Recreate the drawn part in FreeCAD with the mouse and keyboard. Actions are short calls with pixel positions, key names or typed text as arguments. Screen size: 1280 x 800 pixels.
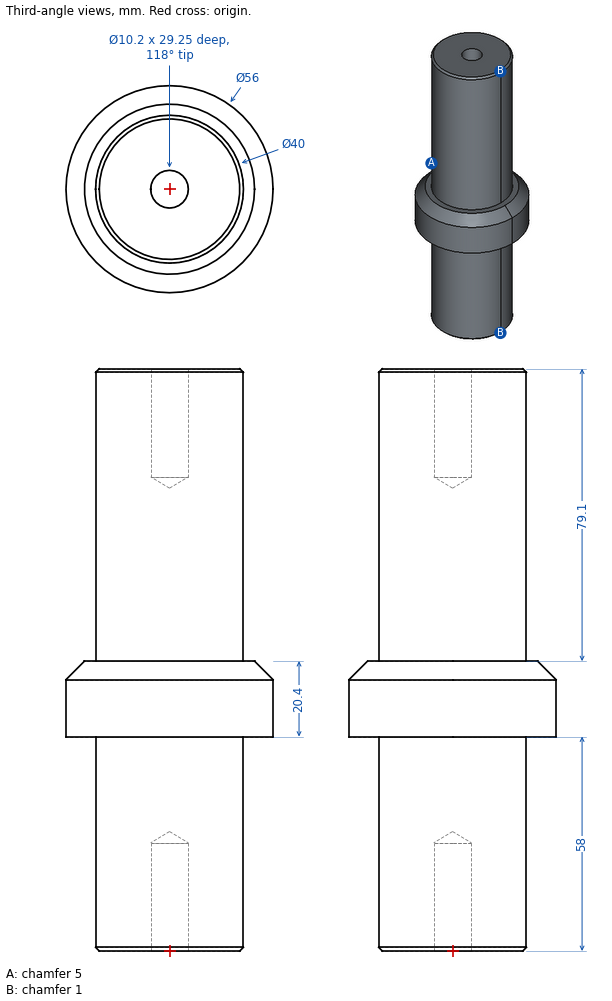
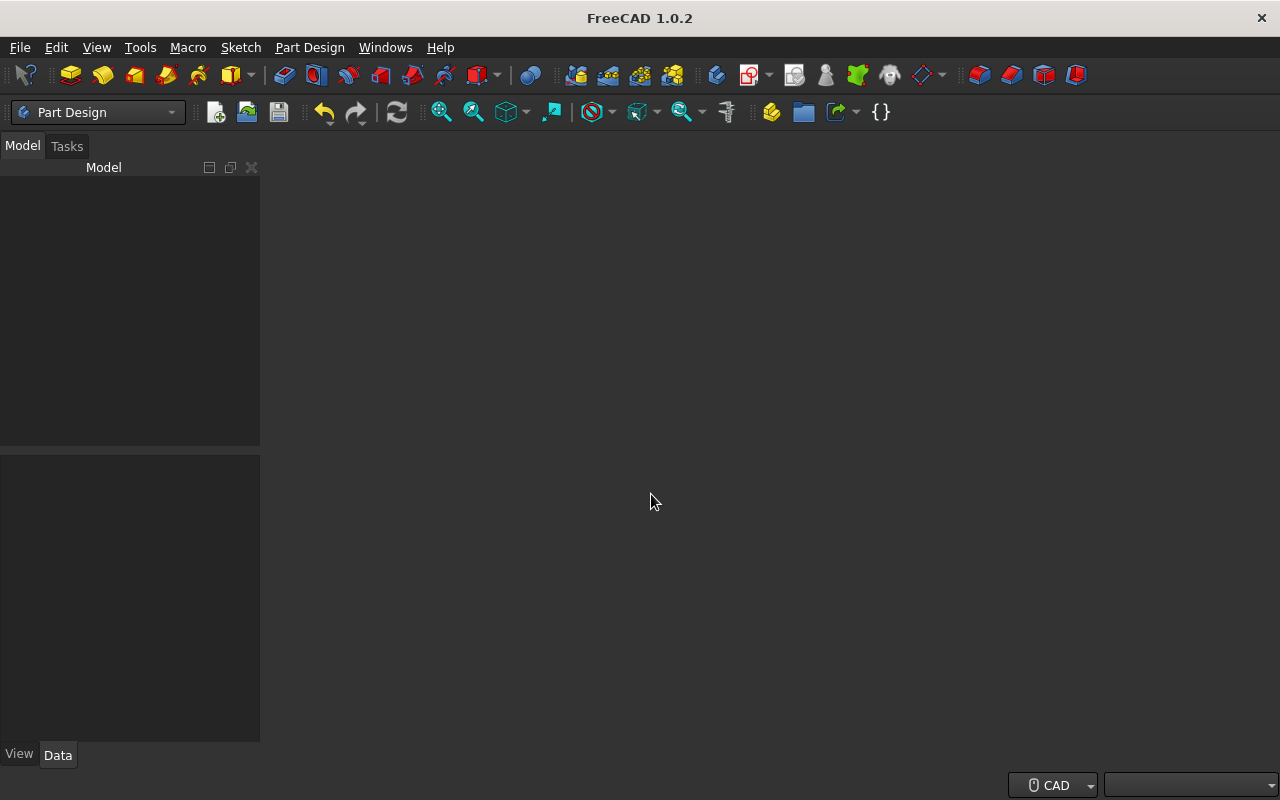
click(216, 112)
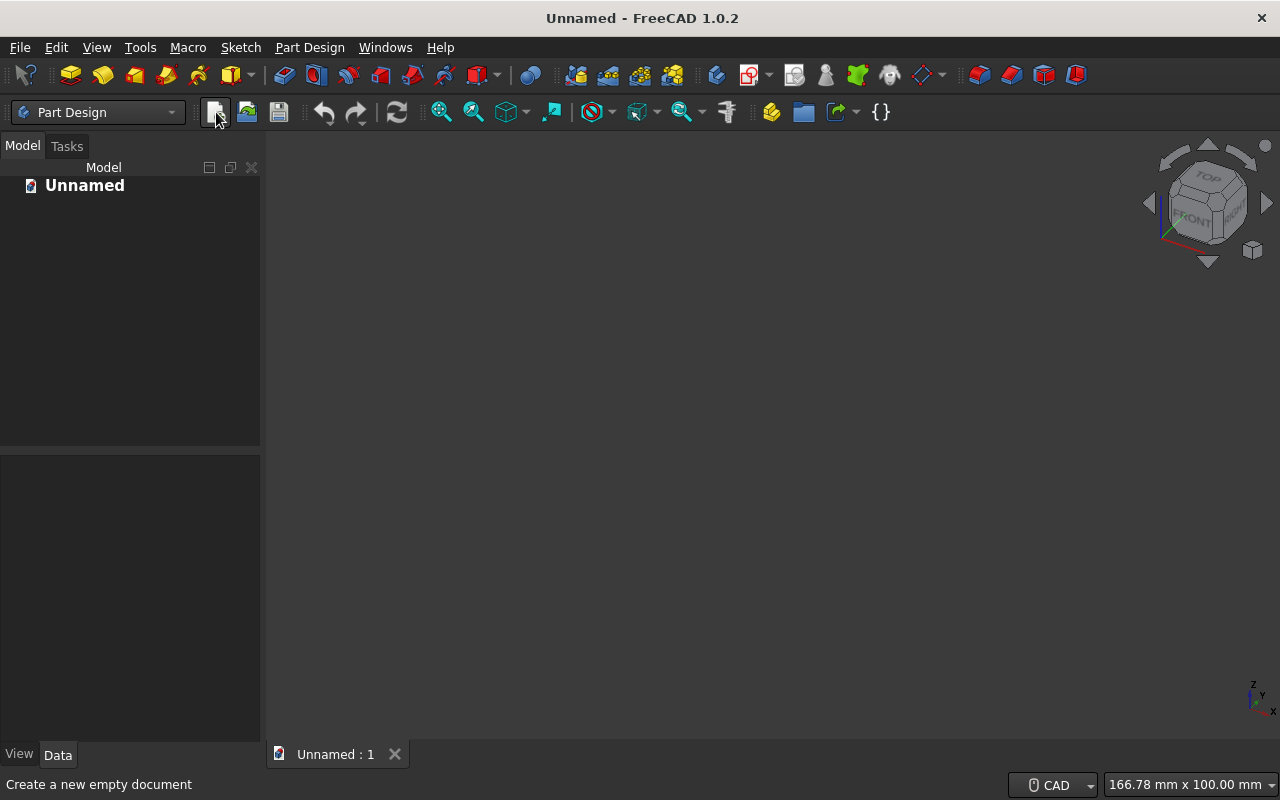
click(750, 76)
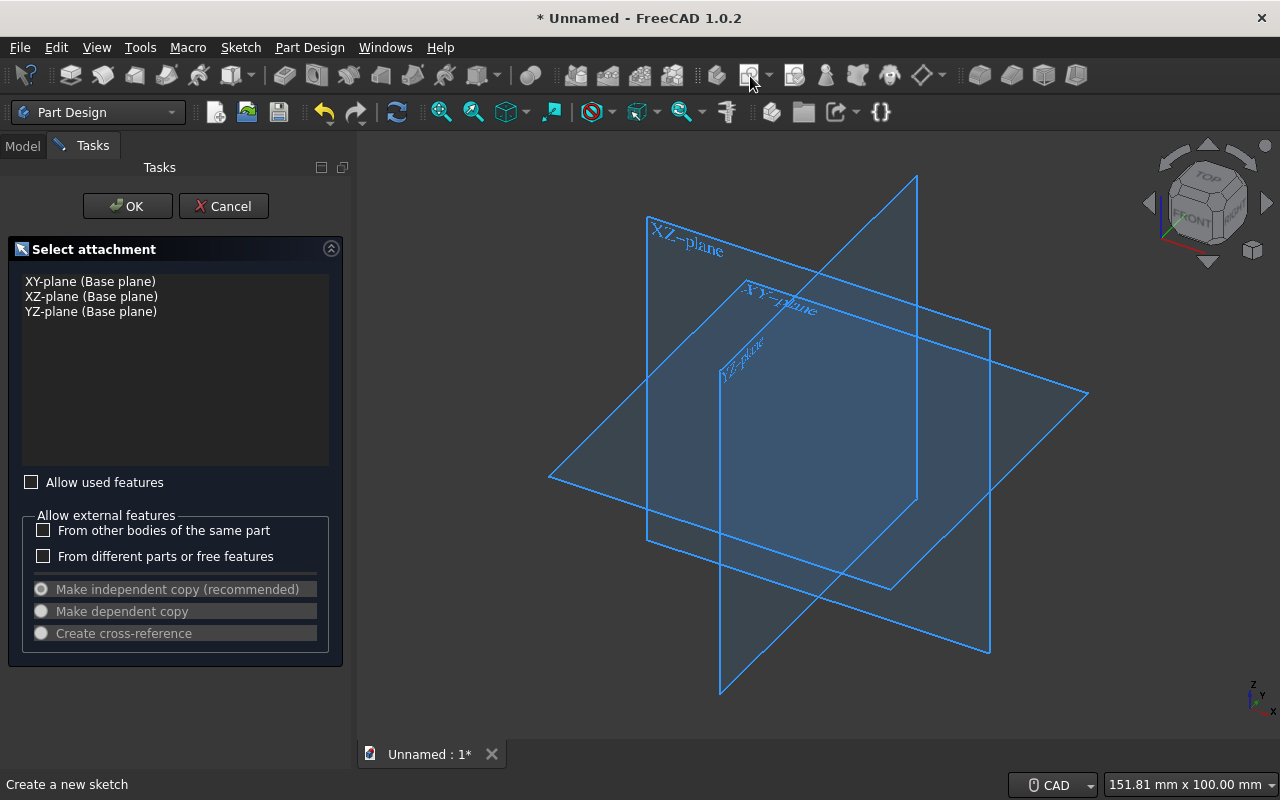
click(82, 282)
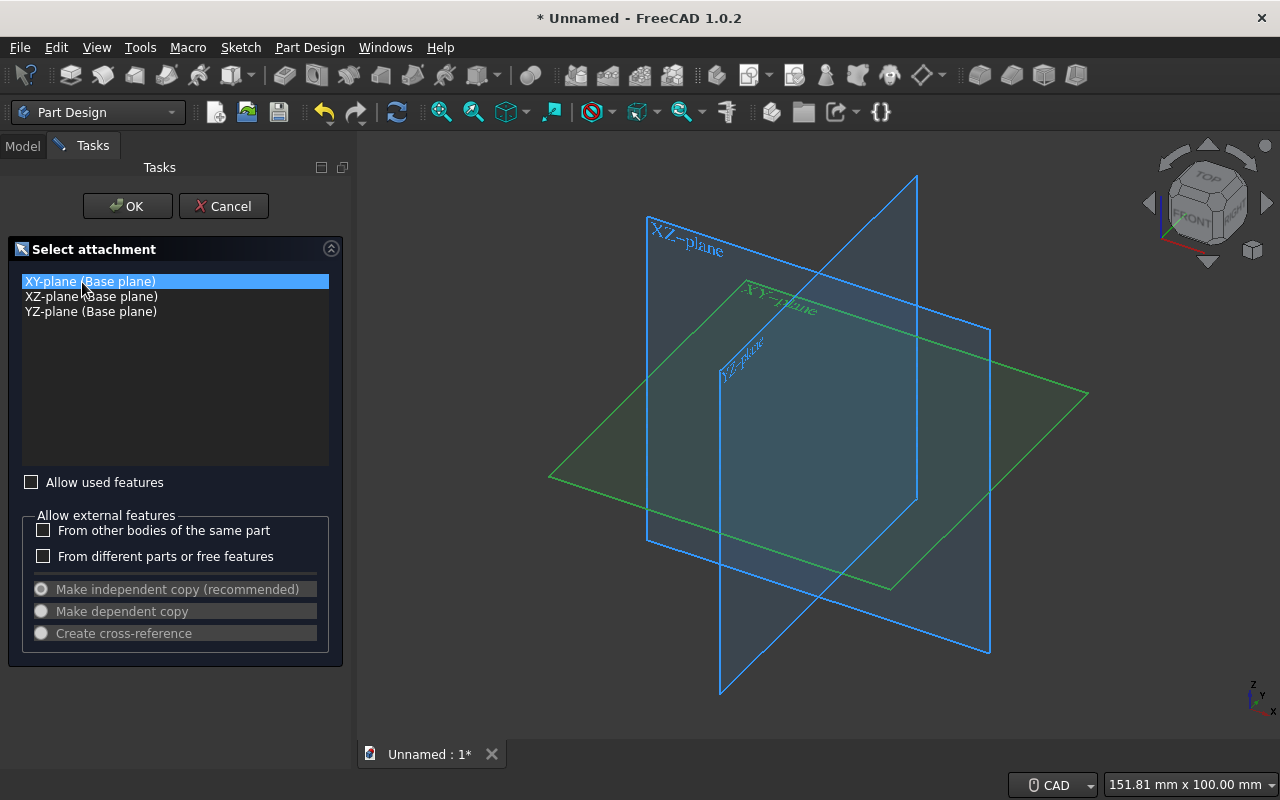
click(128, 206)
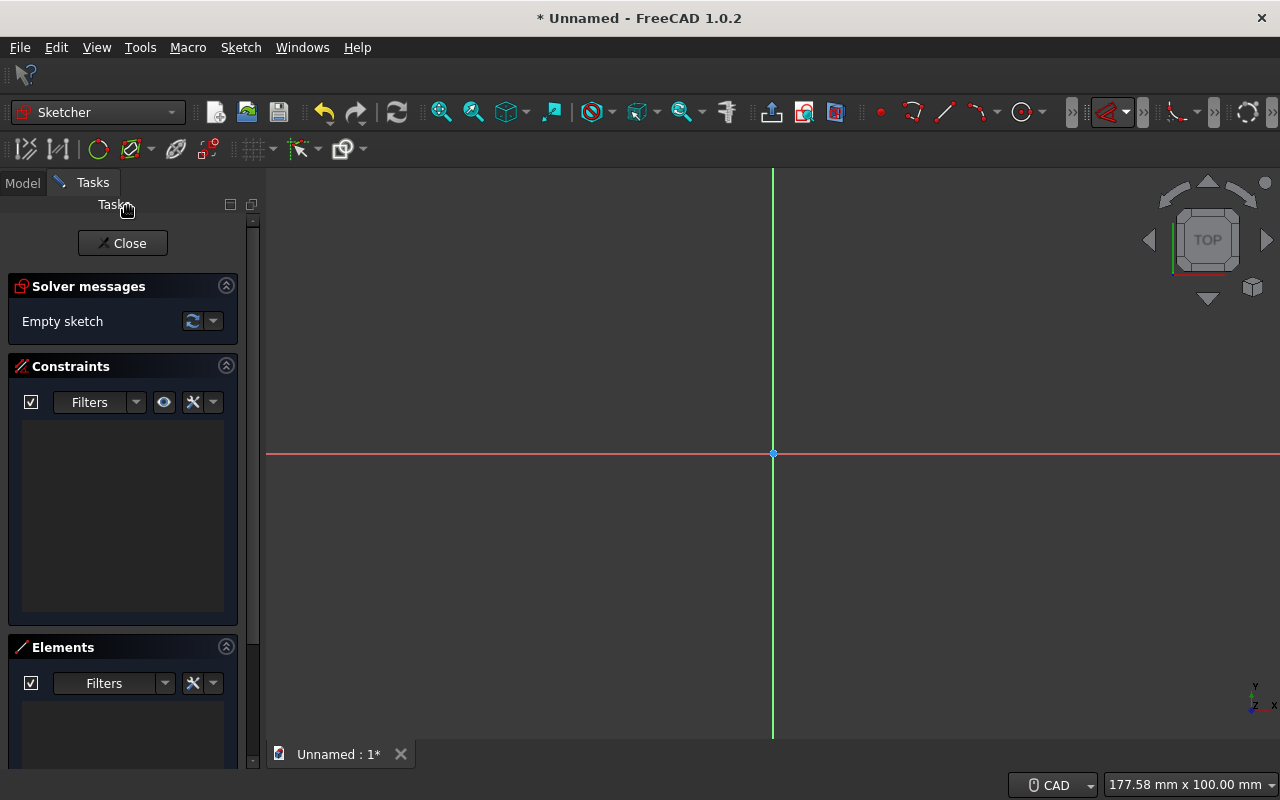
scroll(912, 454, up, 2)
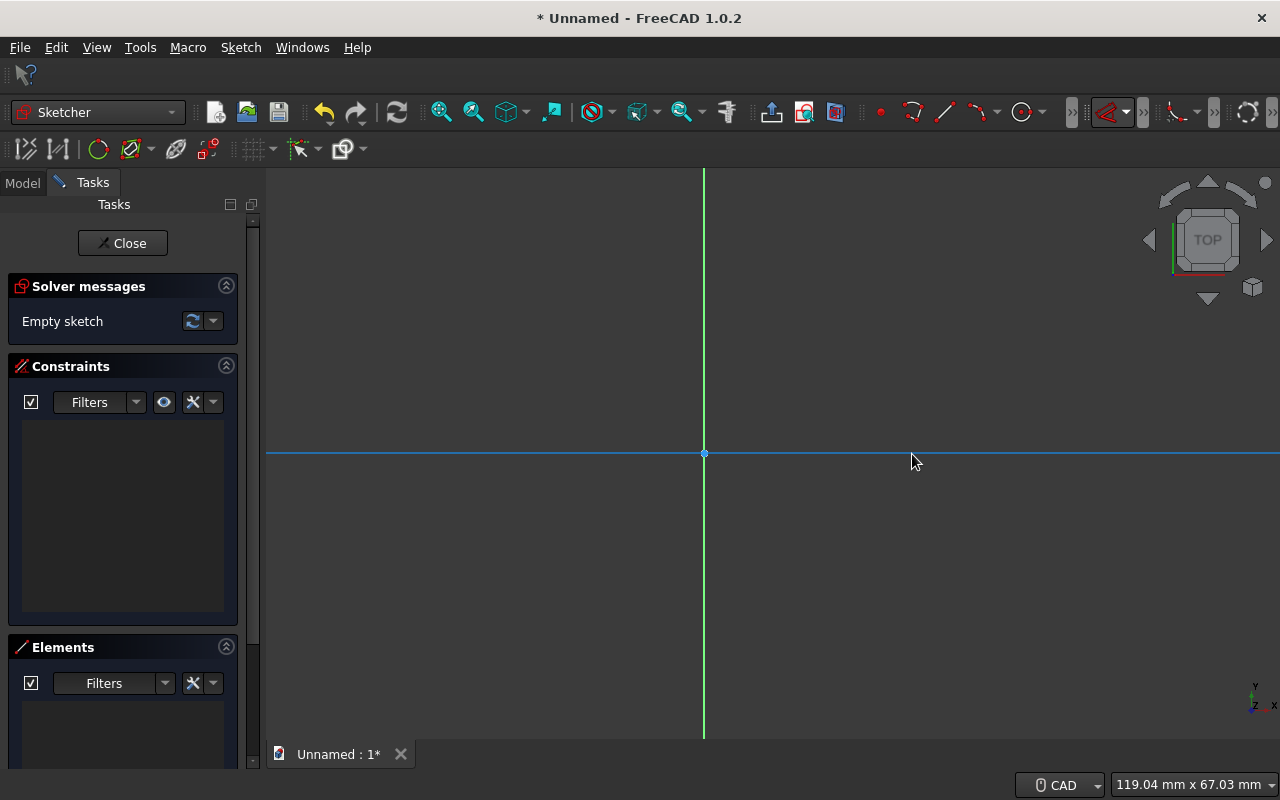
click(1022, 112)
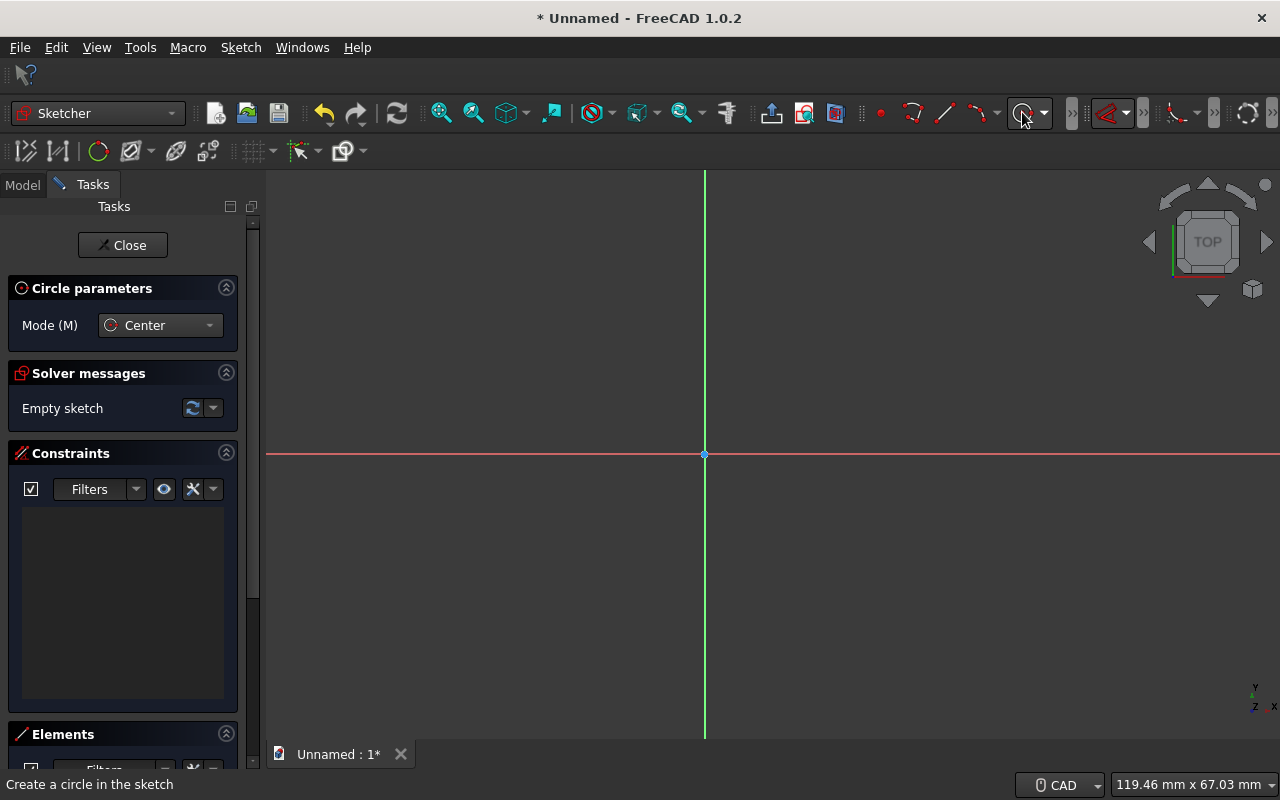
click(705, 454)
move(825, 334)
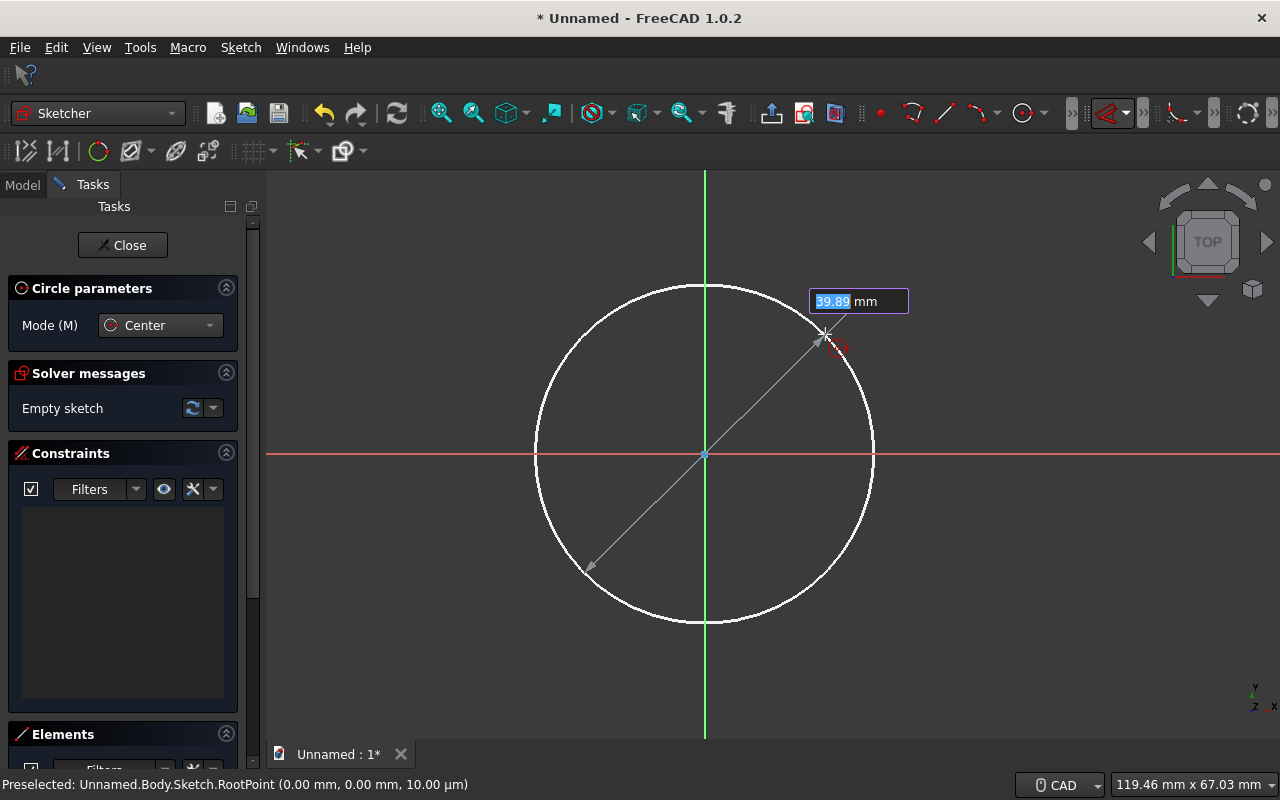
text(40)
key(Return)
key(Escape)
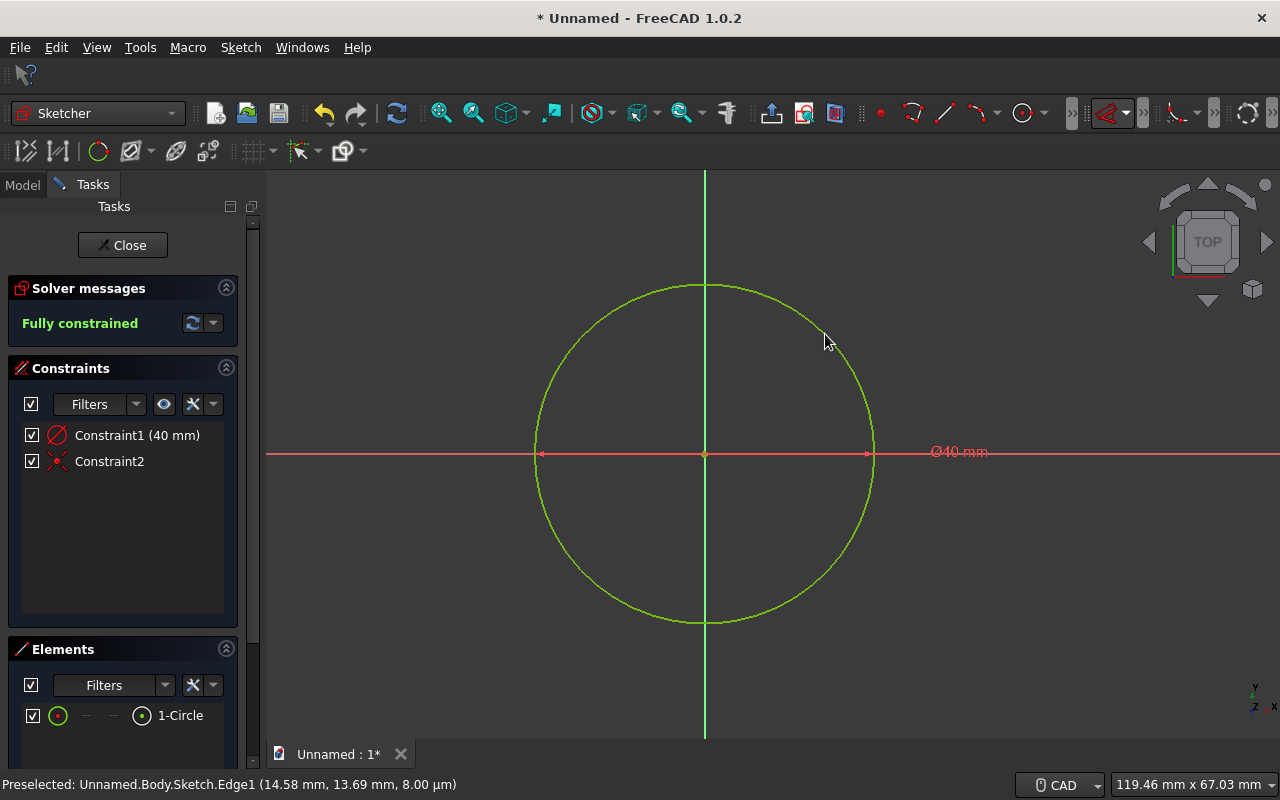
click(123, 245)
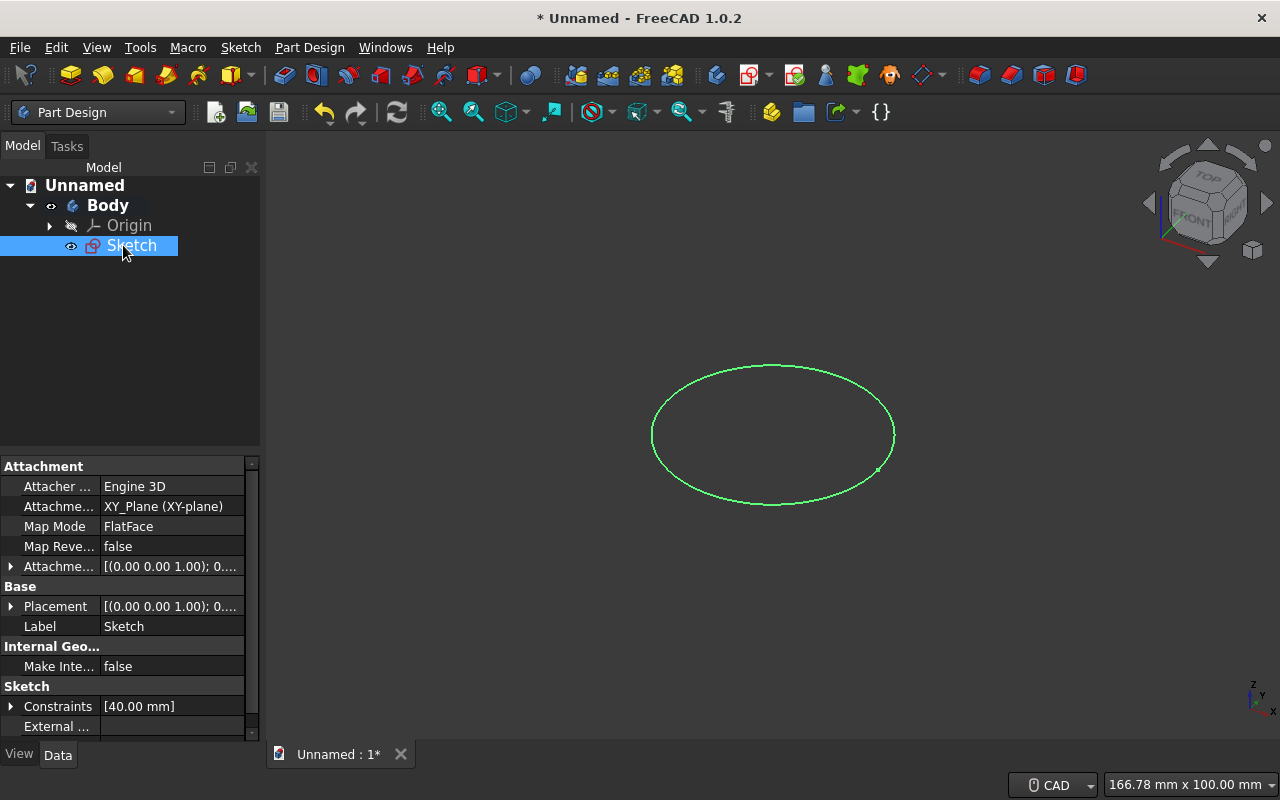
click(72, 76)